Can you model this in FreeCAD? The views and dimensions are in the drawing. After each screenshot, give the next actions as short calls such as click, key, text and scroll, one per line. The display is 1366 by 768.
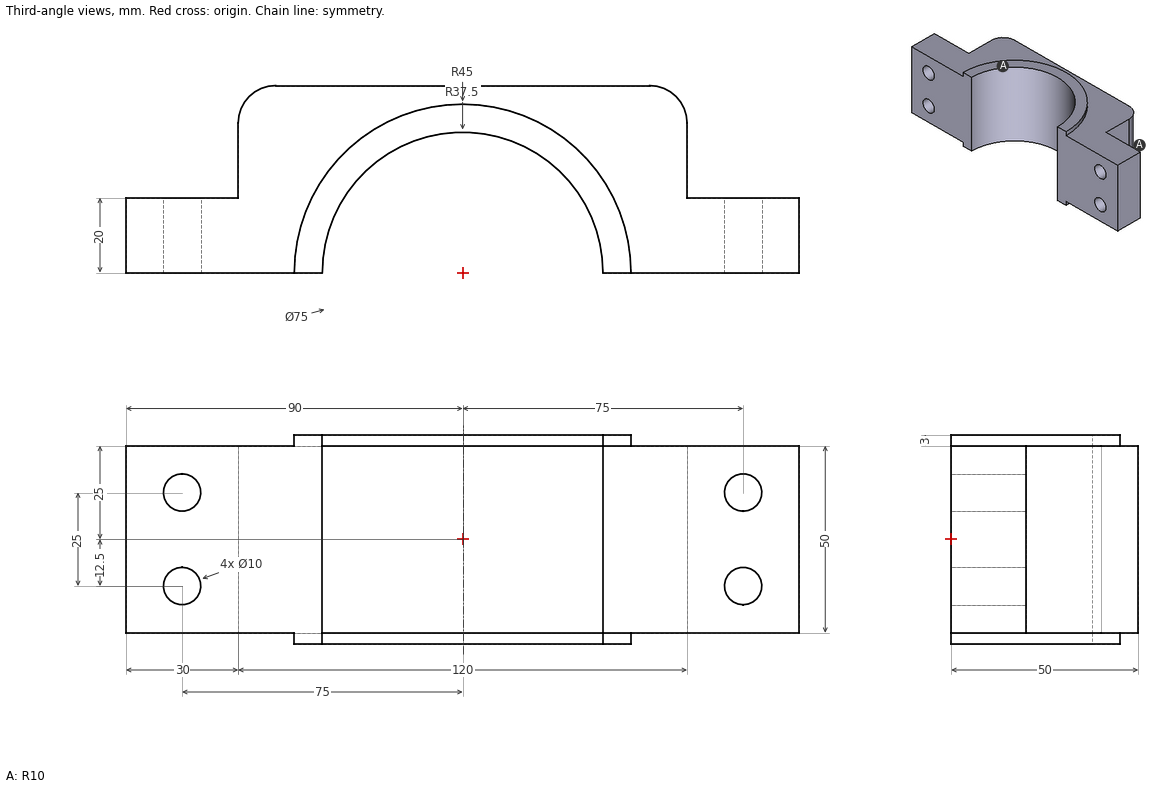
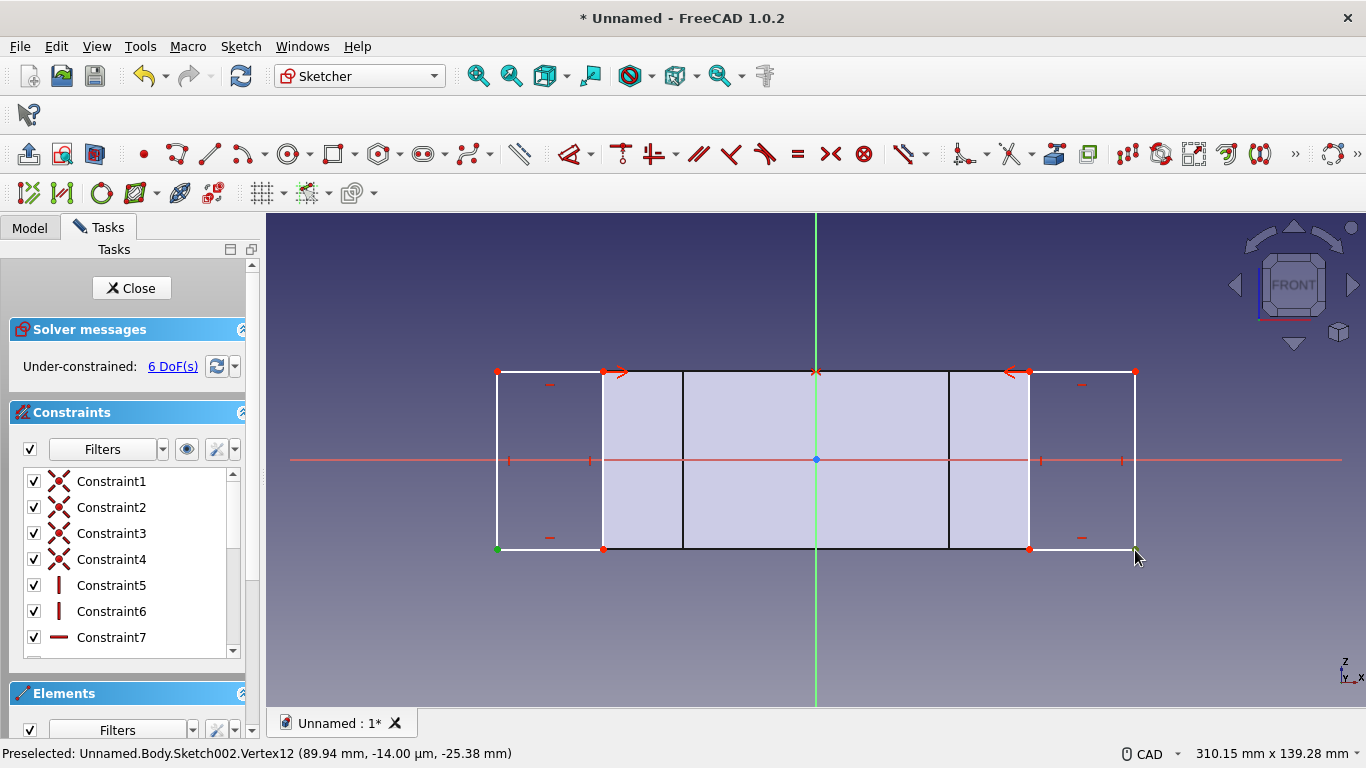
click(816, 648)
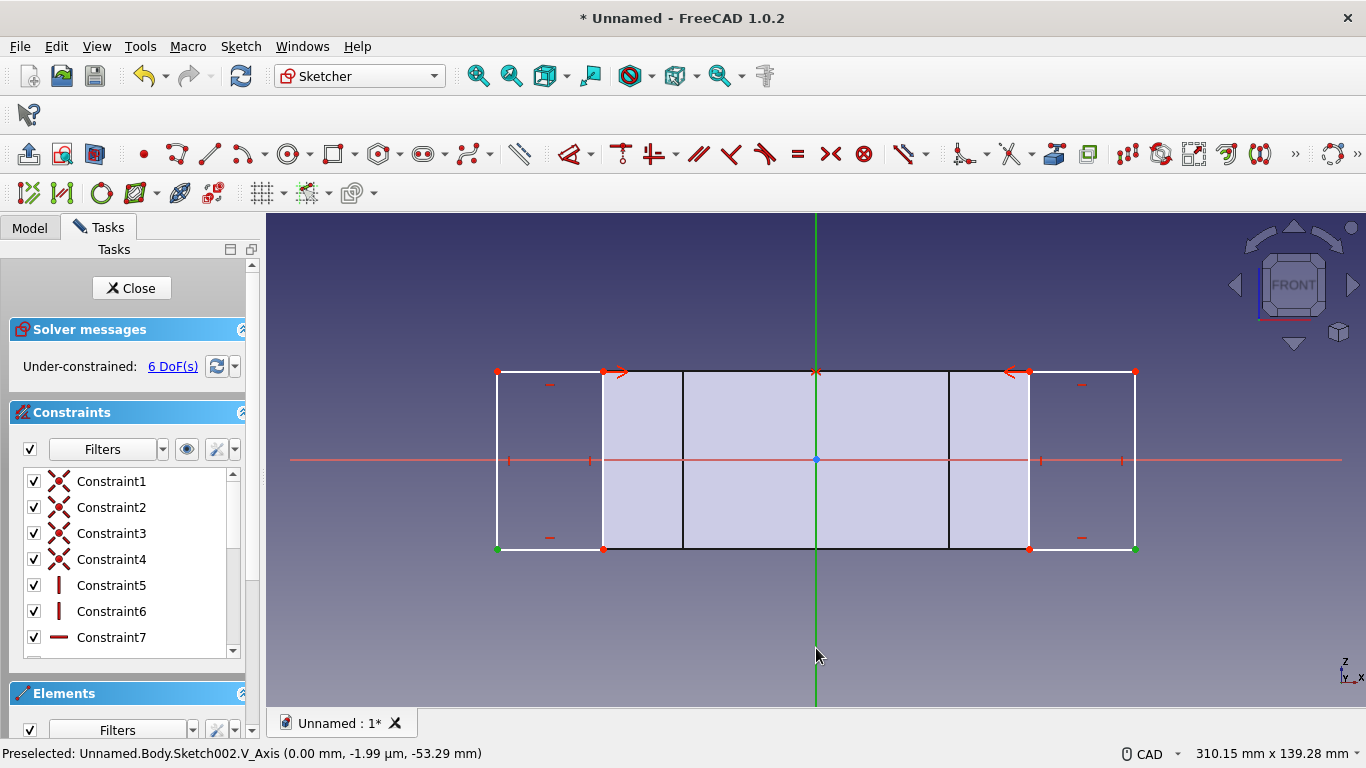
key(s)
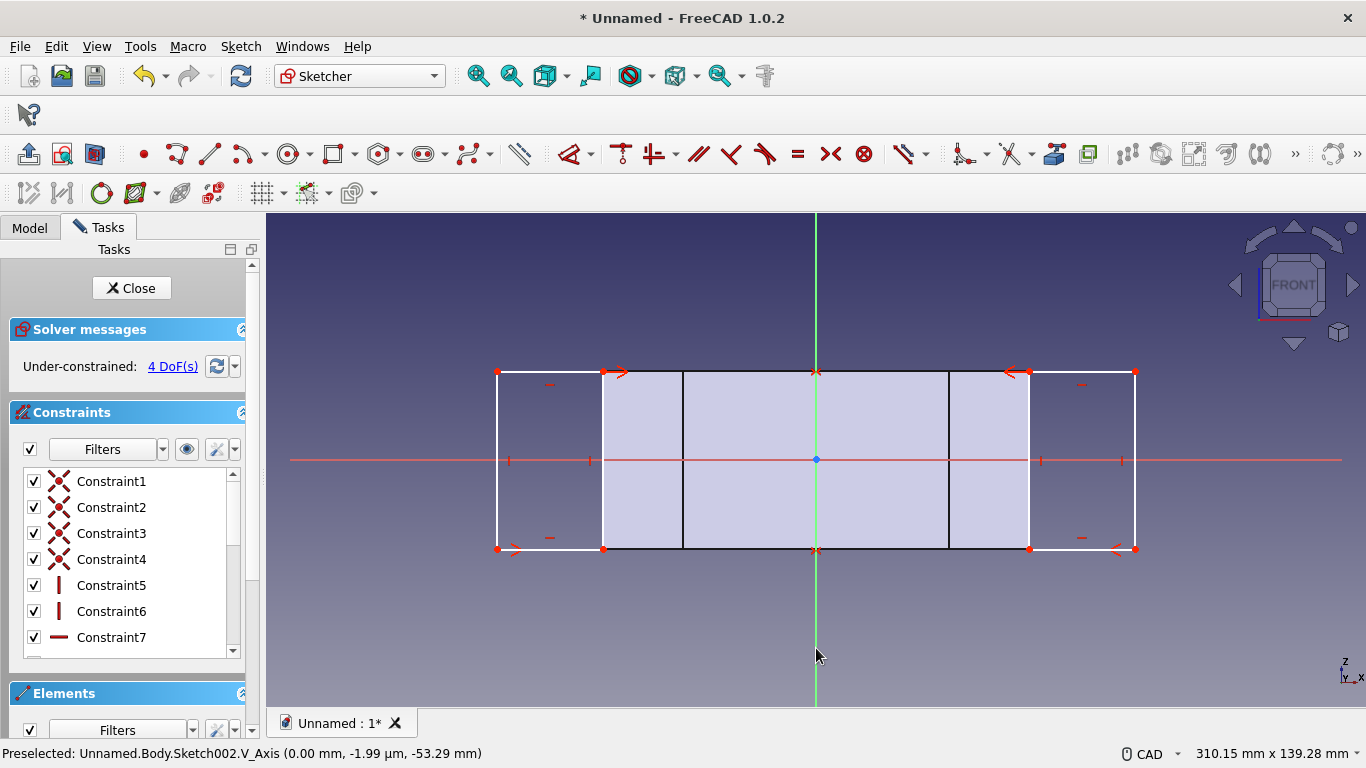
click(497, 425)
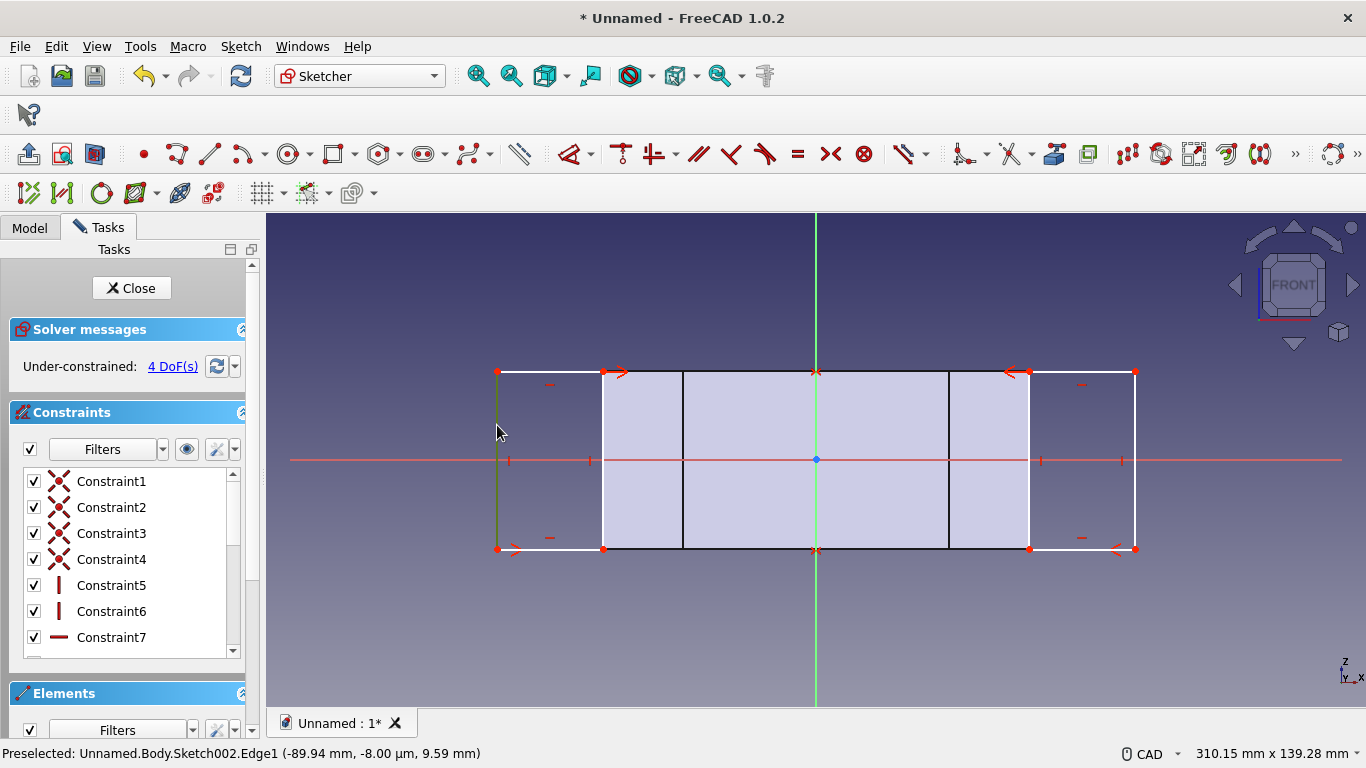
key(i)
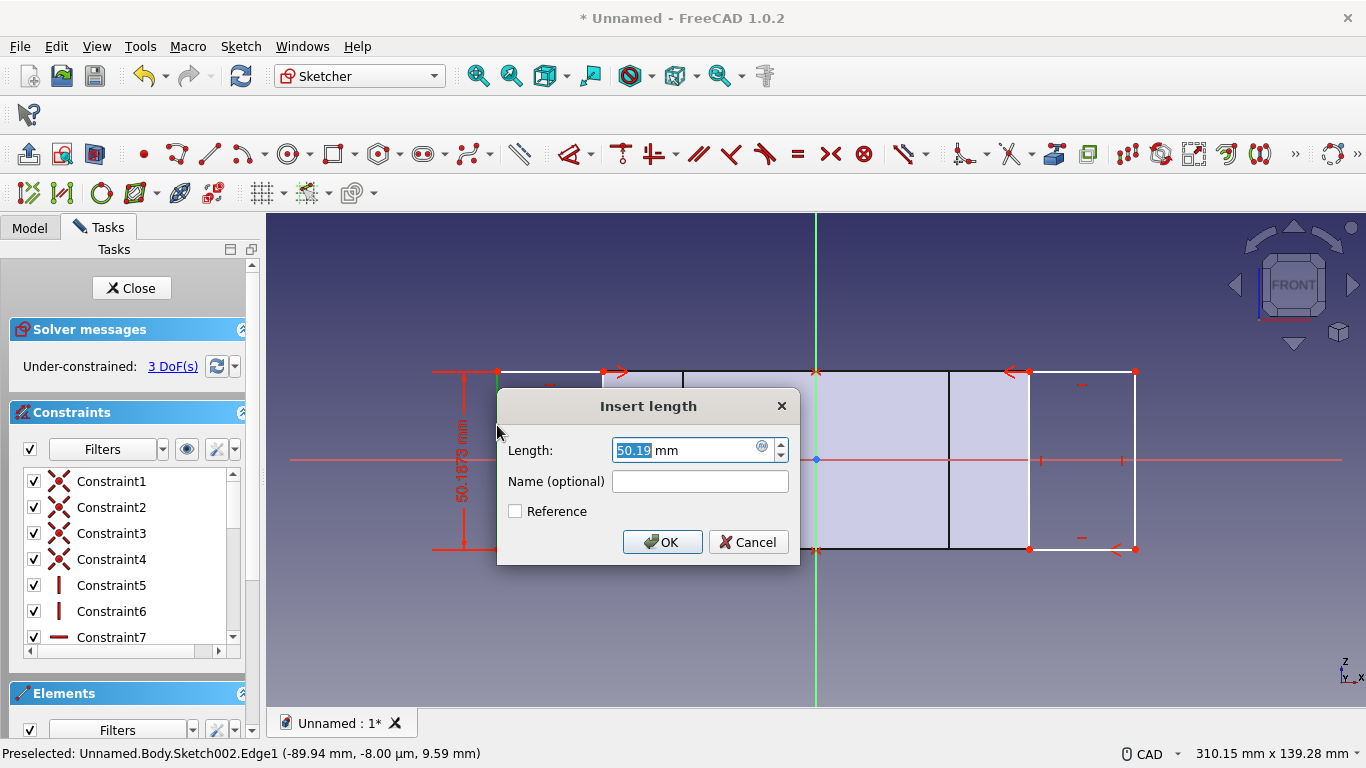
text(50)
key(Return)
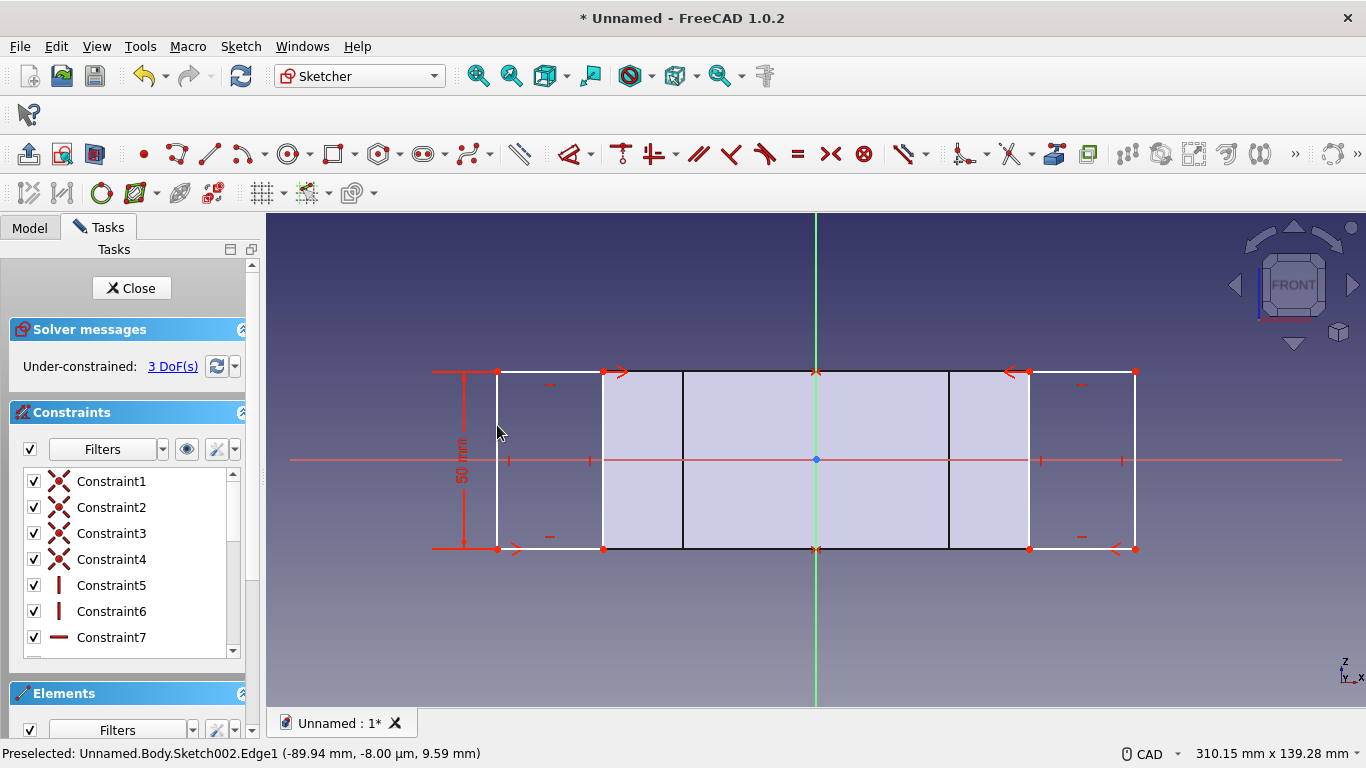
click(529, 549)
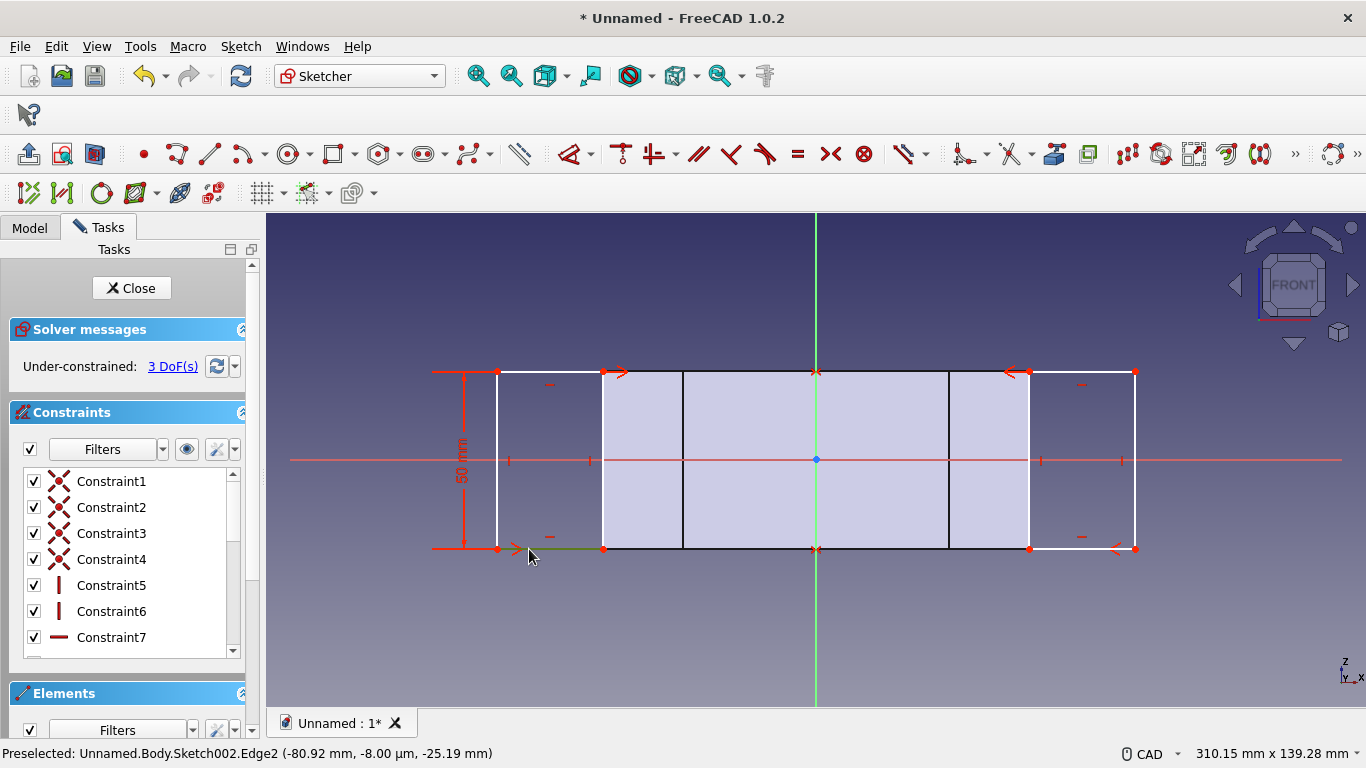
key(l)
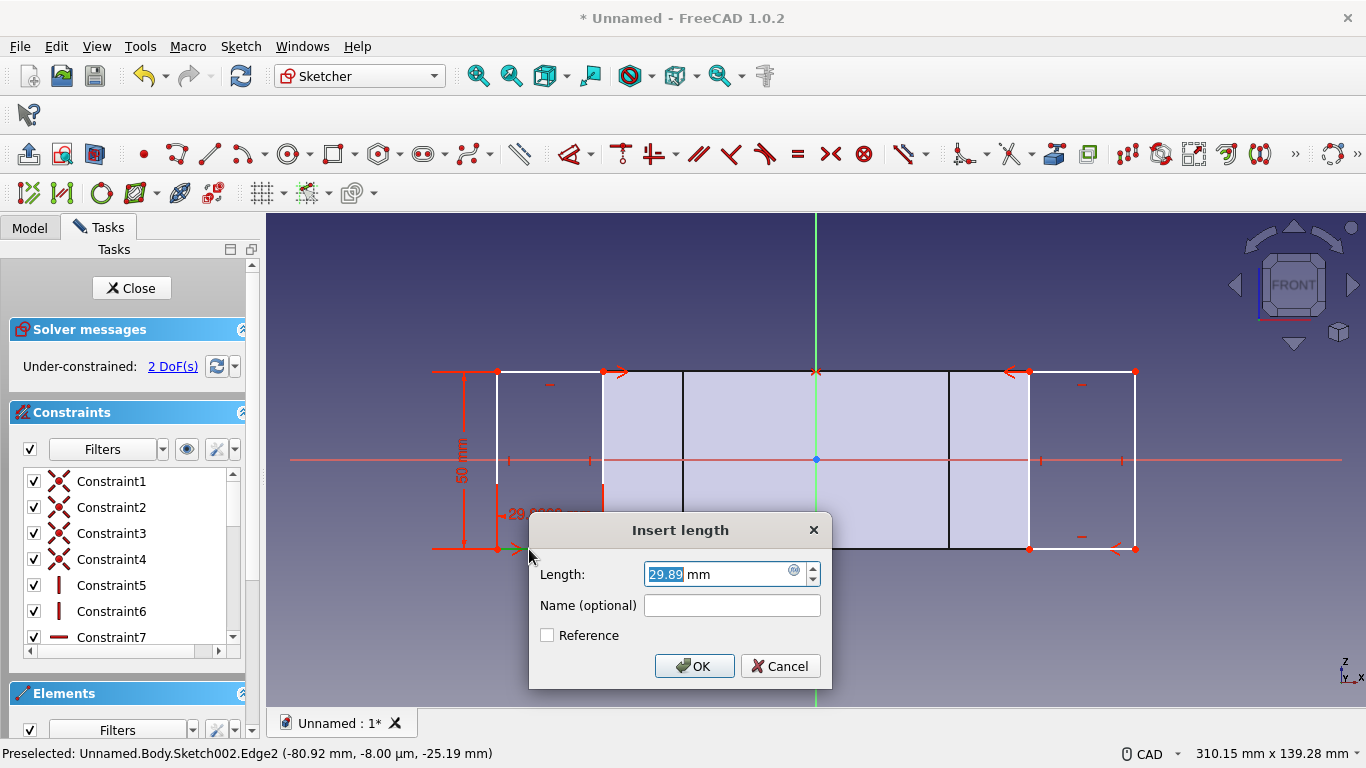
text(30)
key(Return)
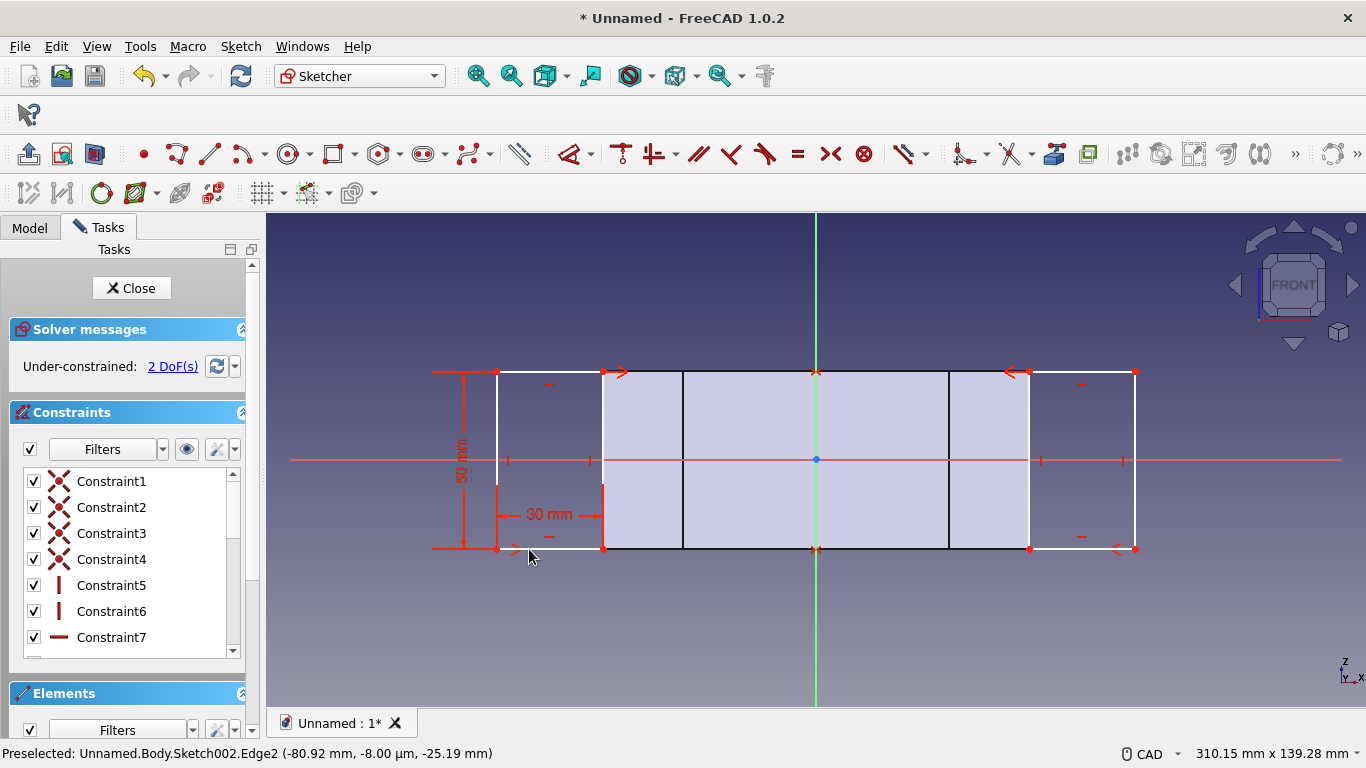
click(497, 372)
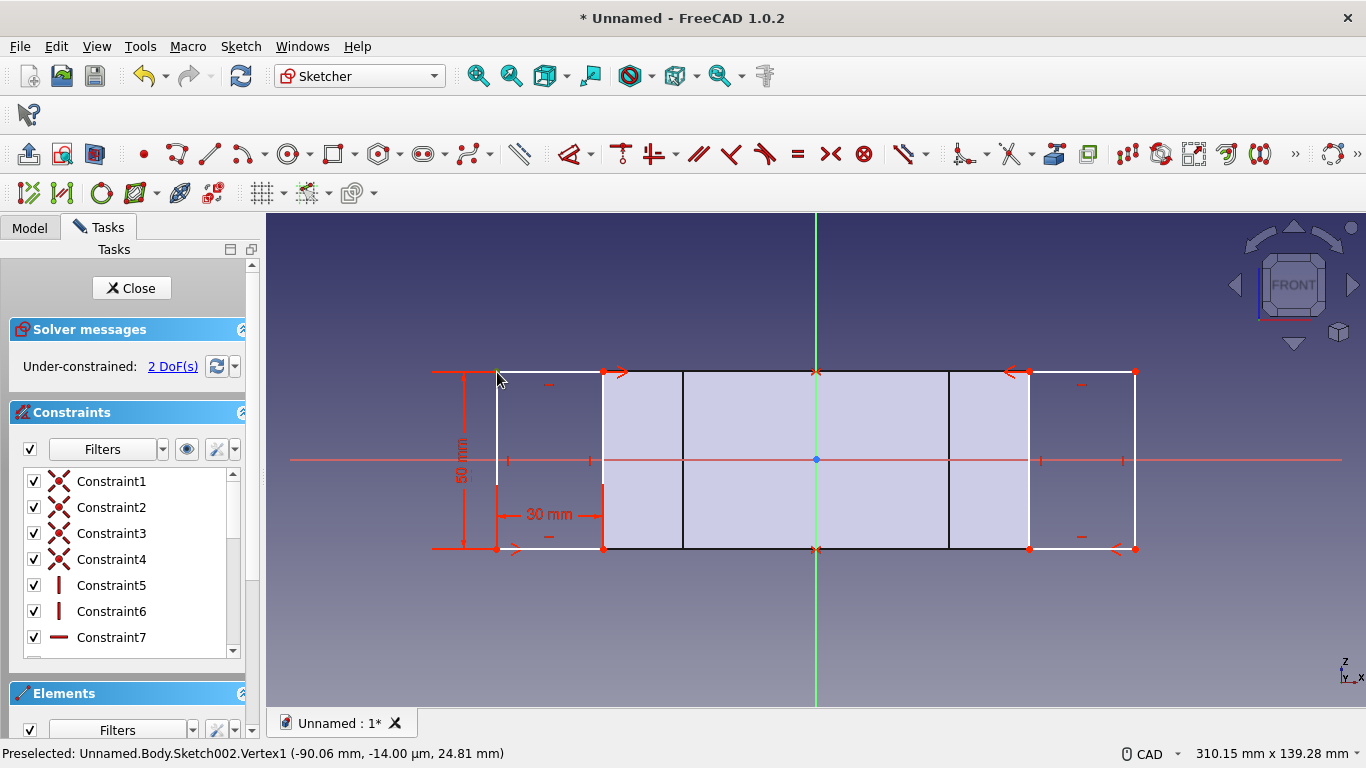
key(l)